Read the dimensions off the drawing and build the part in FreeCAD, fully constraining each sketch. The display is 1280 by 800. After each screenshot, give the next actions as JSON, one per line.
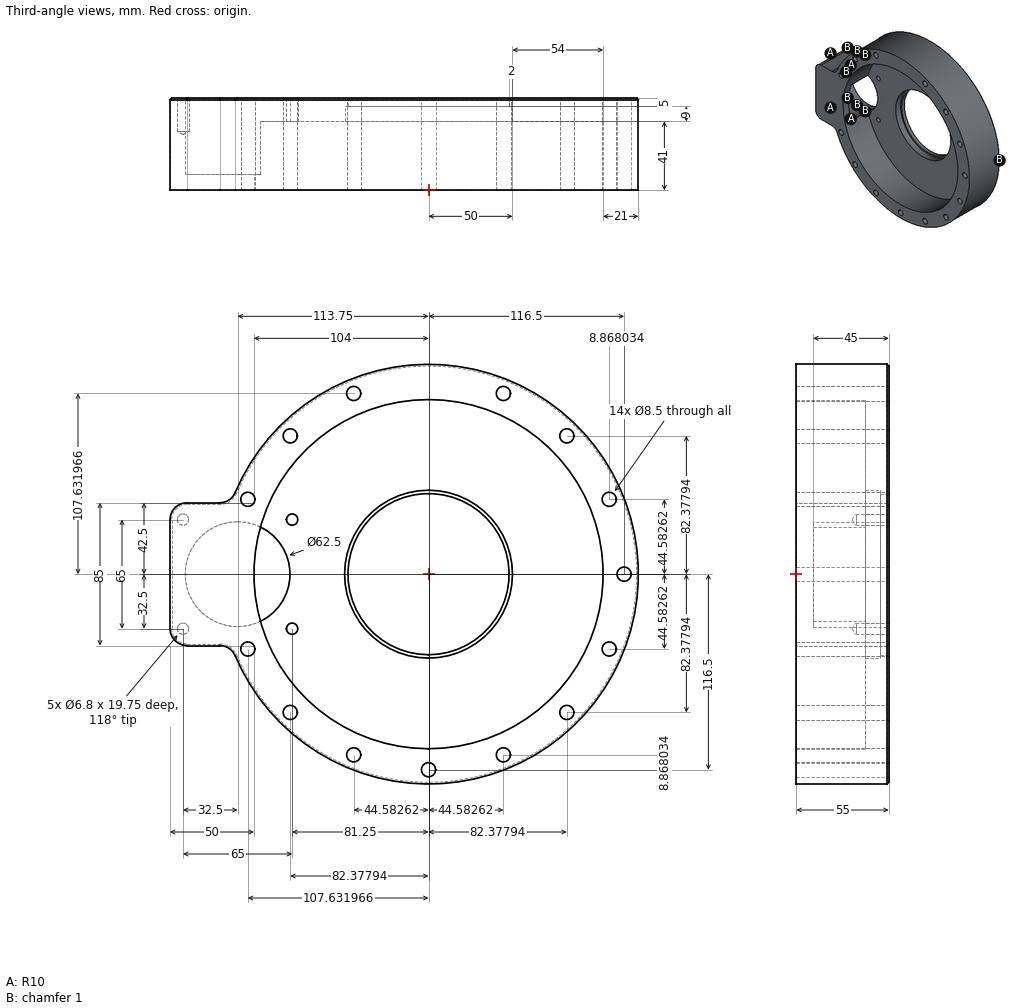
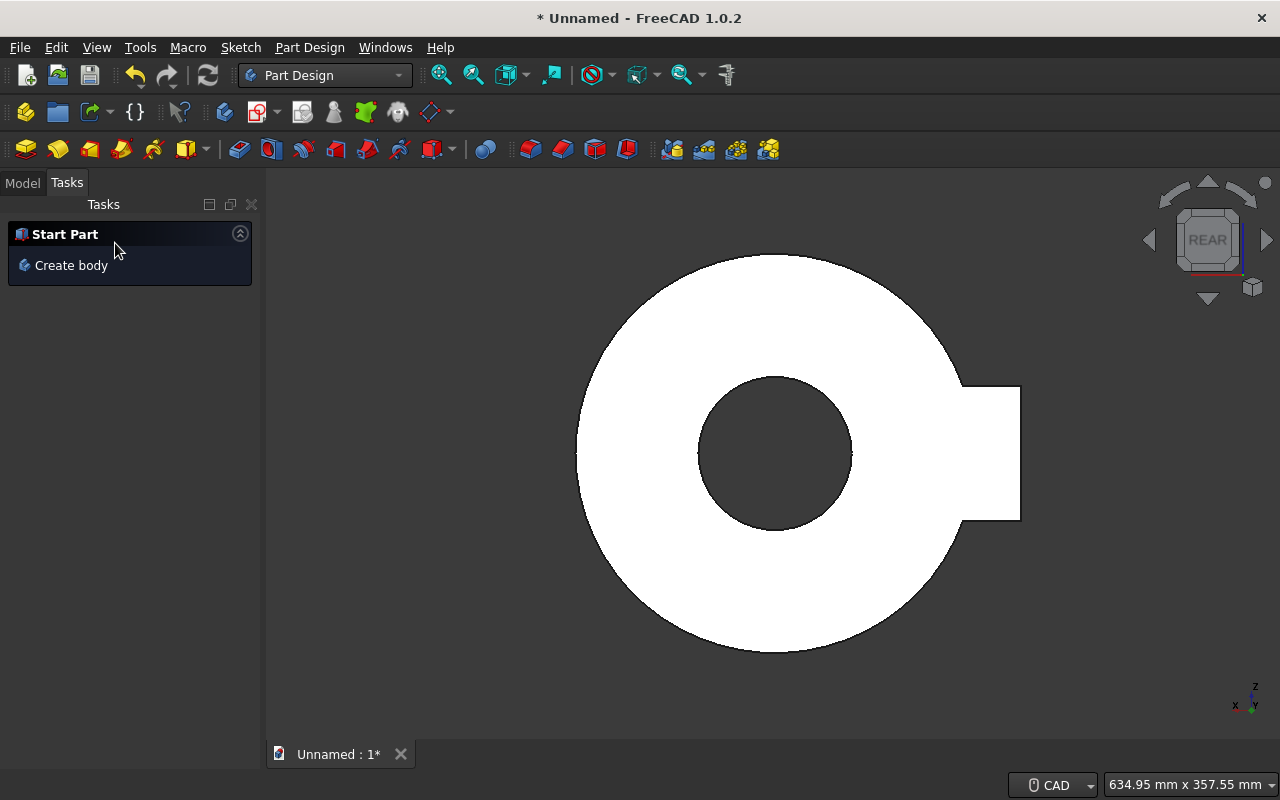
{"action": "left_click", "coordinate": [926, 453]}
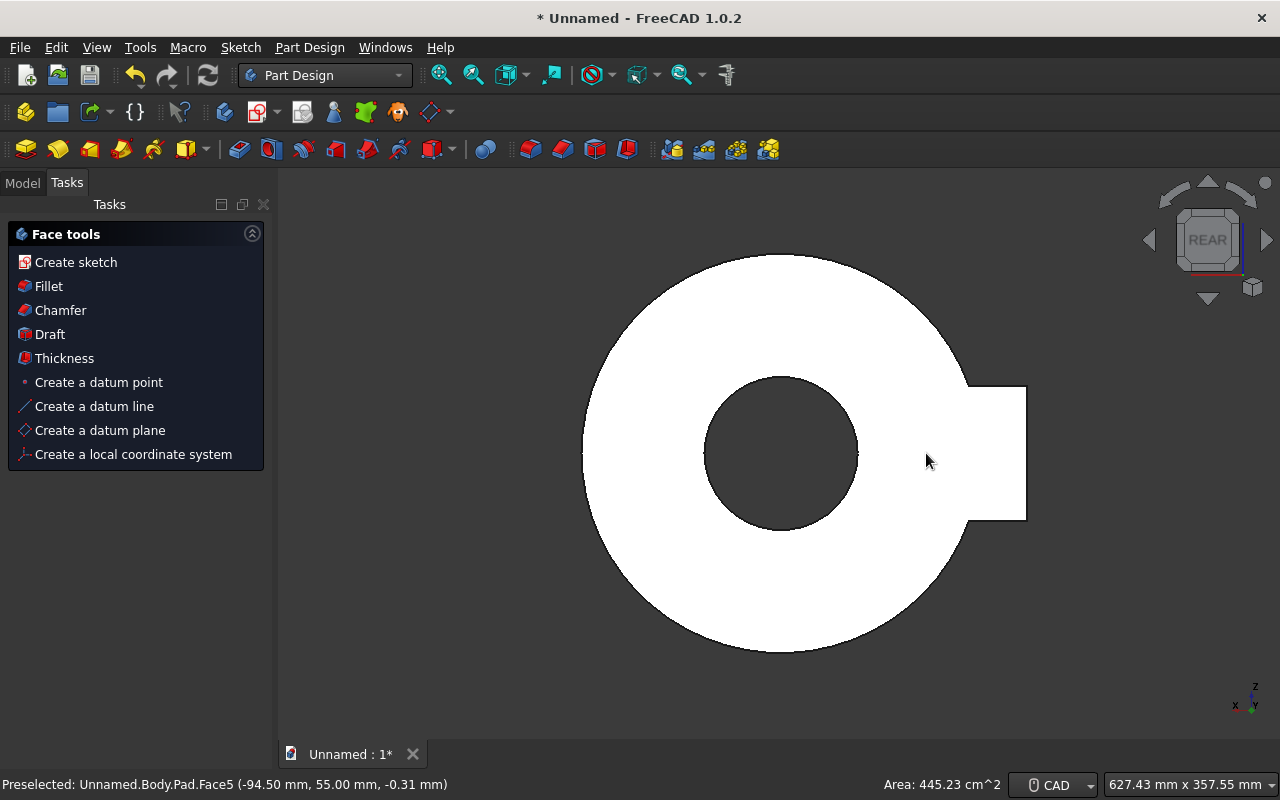
{"action": "left_click", "coordinate": [258, 112]}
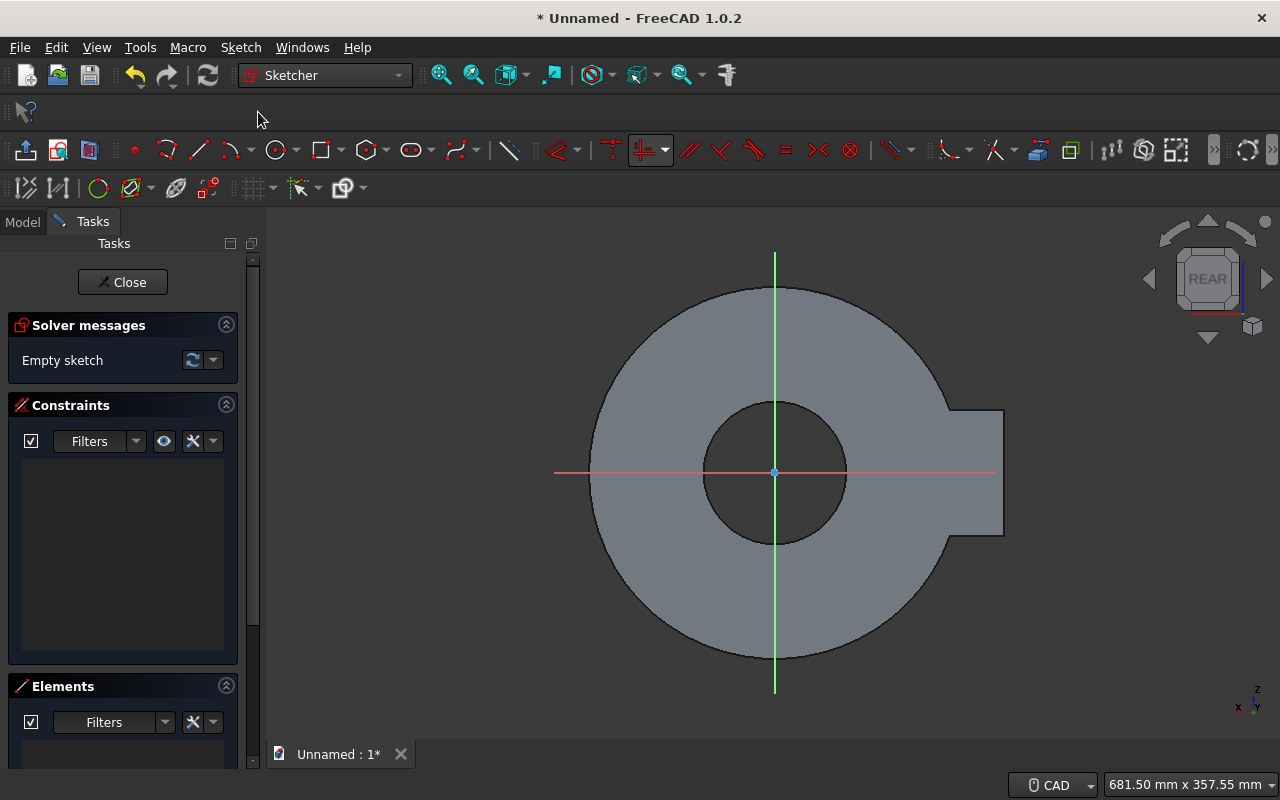
{"action": "scroll", "coordinate": [987, 473], "scroll_direction": "up", "scroll_amount": 5}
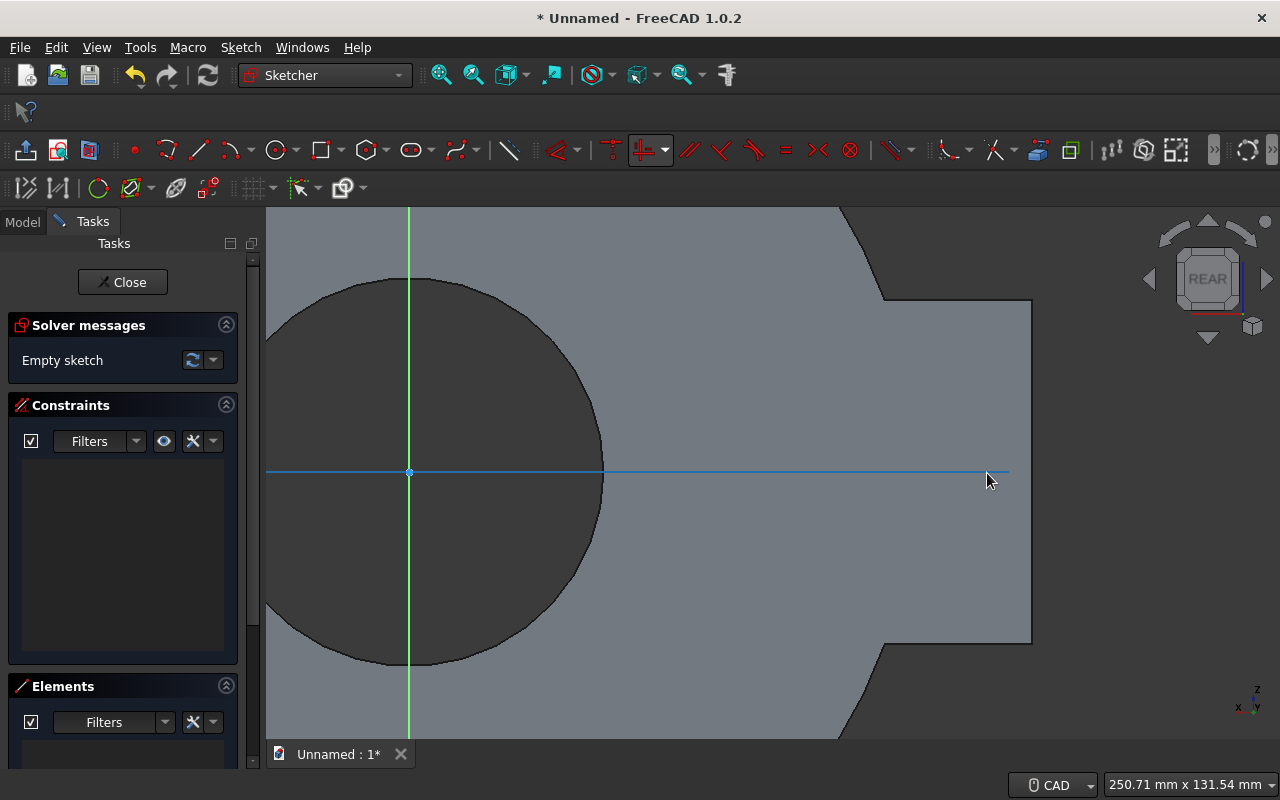
{"action": "left_click", "coordinate": [276, 150]}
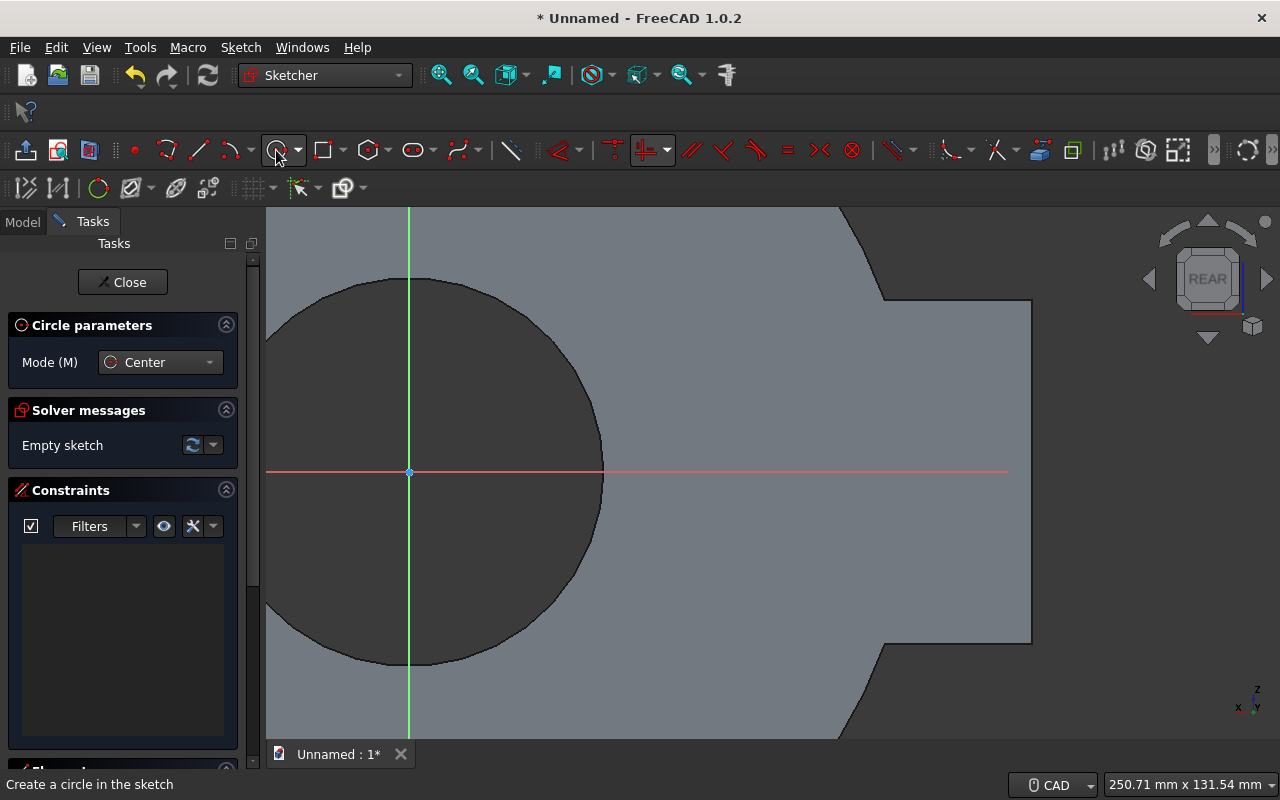
{"action": "left_click", "coordinate": [869, 472]}
{"action": "left_click", "coordinate": [959, 383]}
{"action": "key", "text": "Escape"}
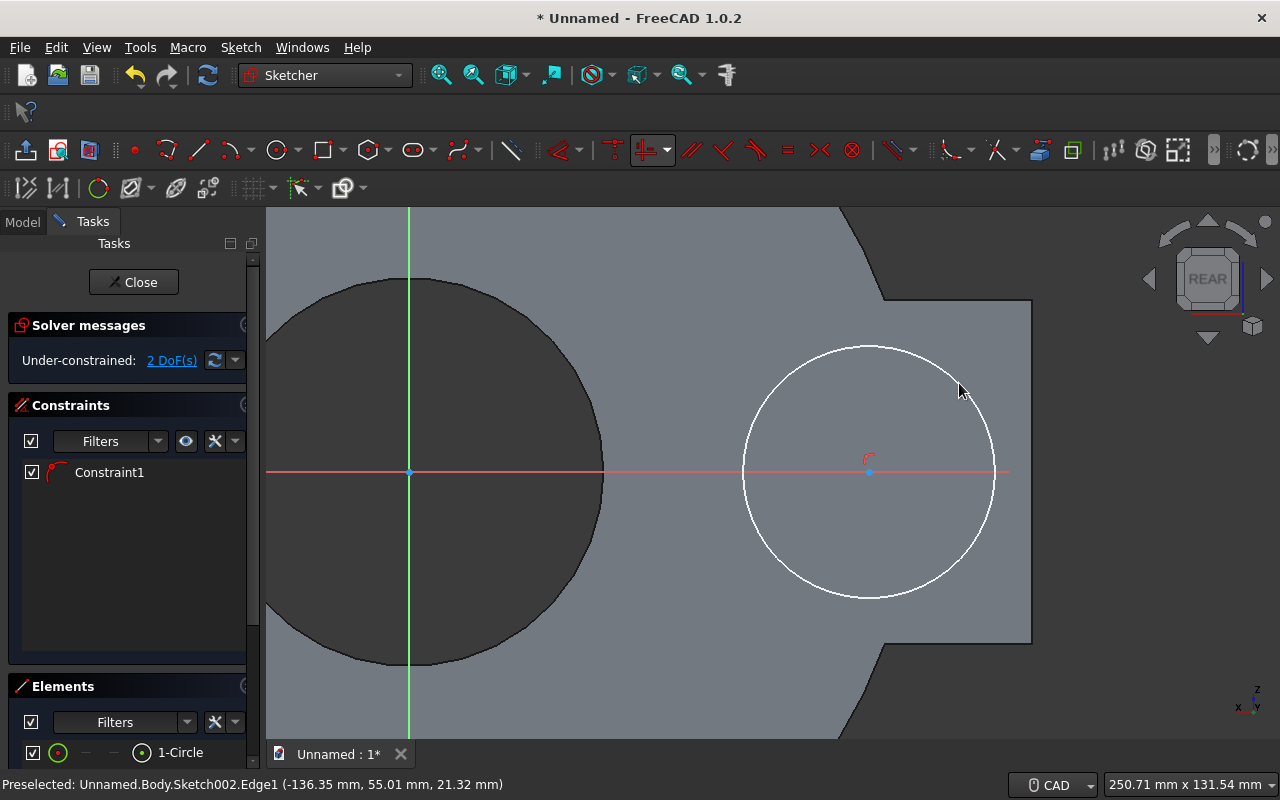
{"action": "left_click", "coordinate": [558, 150]}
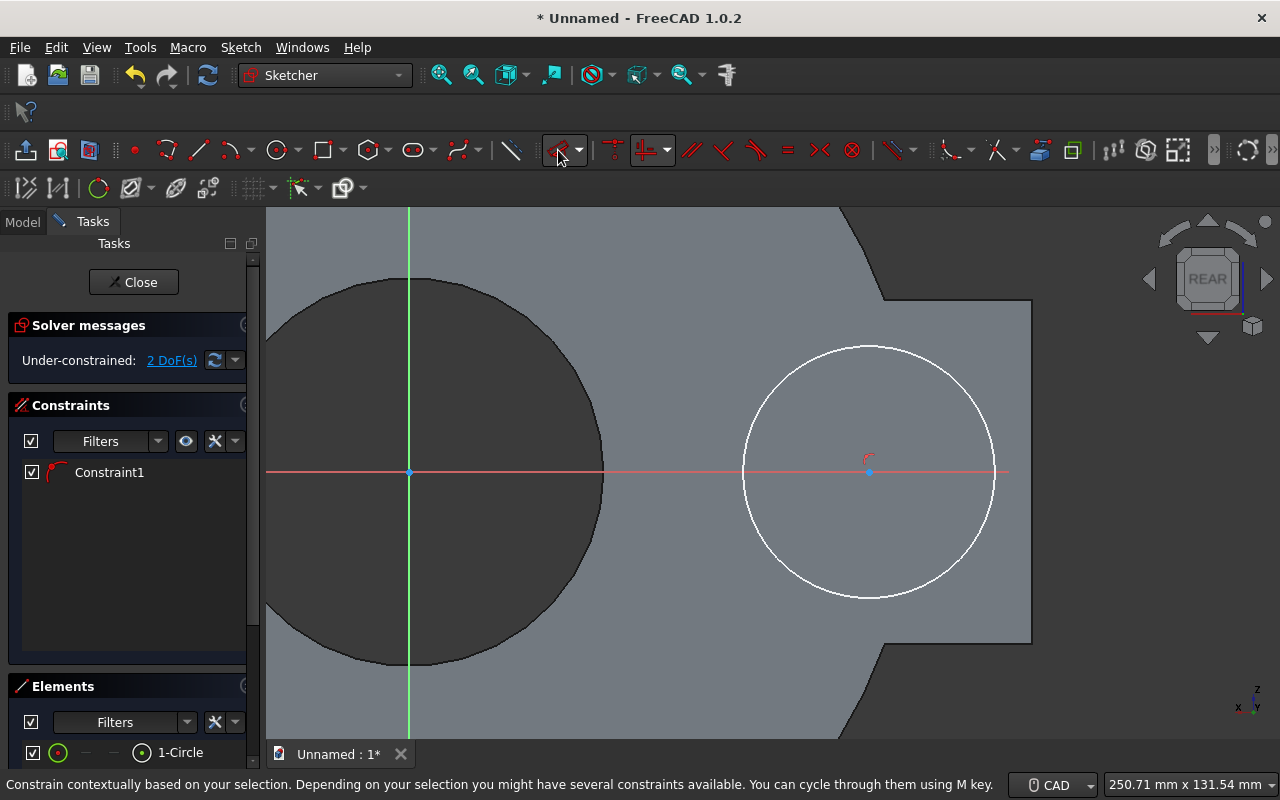
{"action": "left_click", "coordinate": [958, 383]}
{"action": "left_click", "coordinate": [981, 360]}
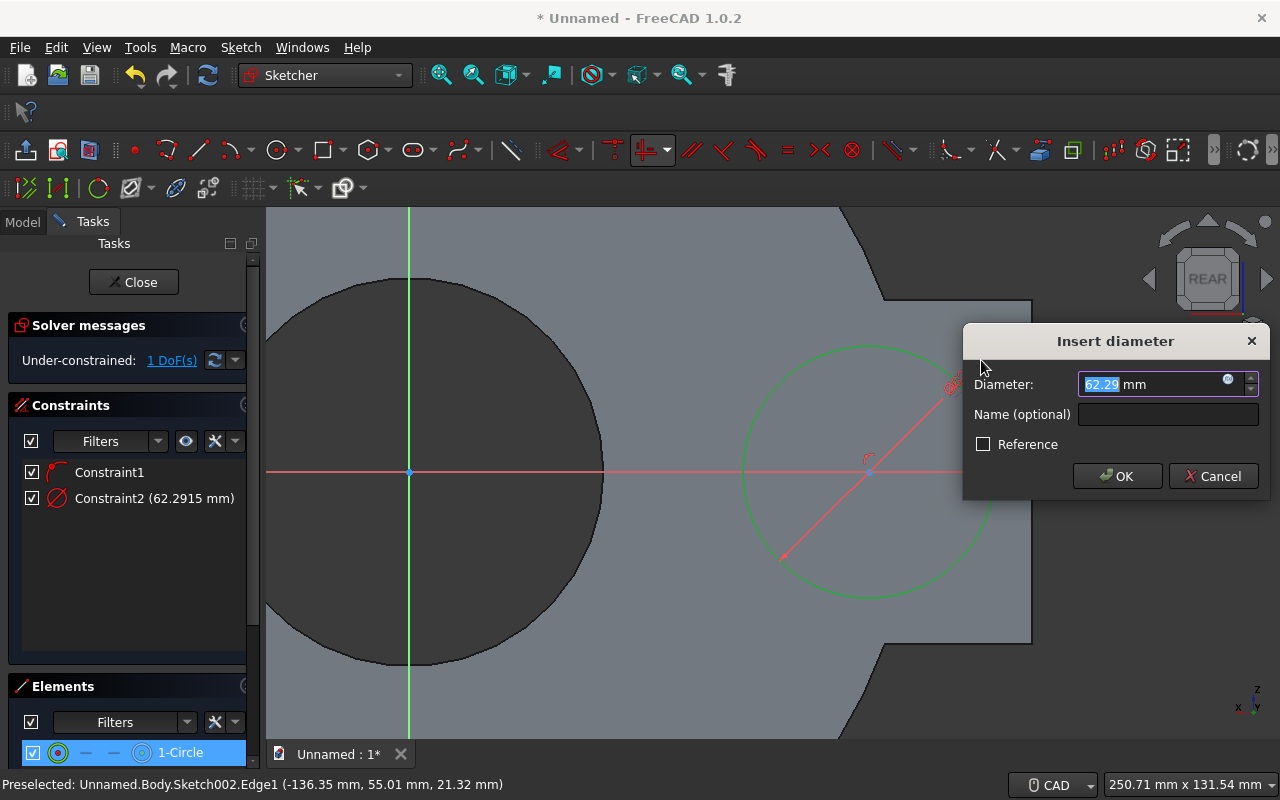
{"action": "type", "text": "62.5"}
{"action": "key", "text": "Return"}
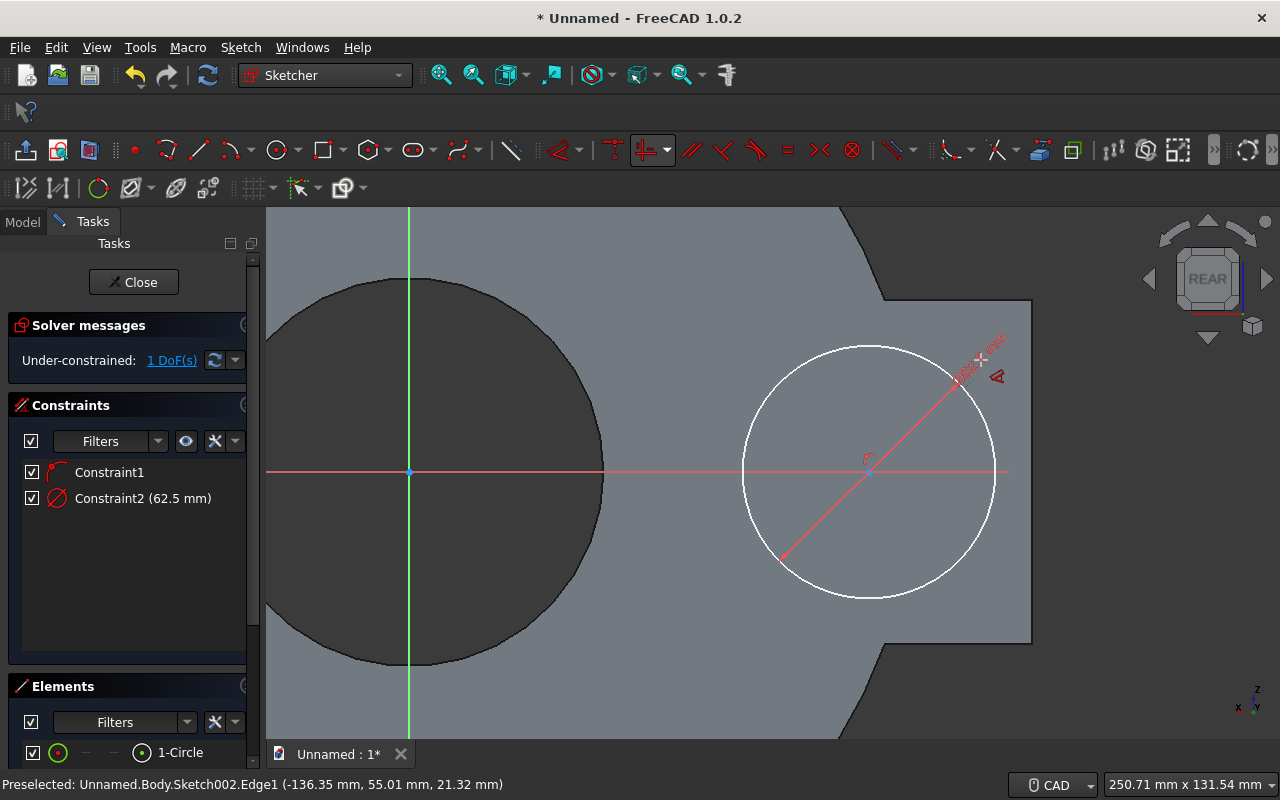
{"action": "left_click", "coordinate": [869, 472]}
{"action": "left_click", "coordinate": [639, 506]}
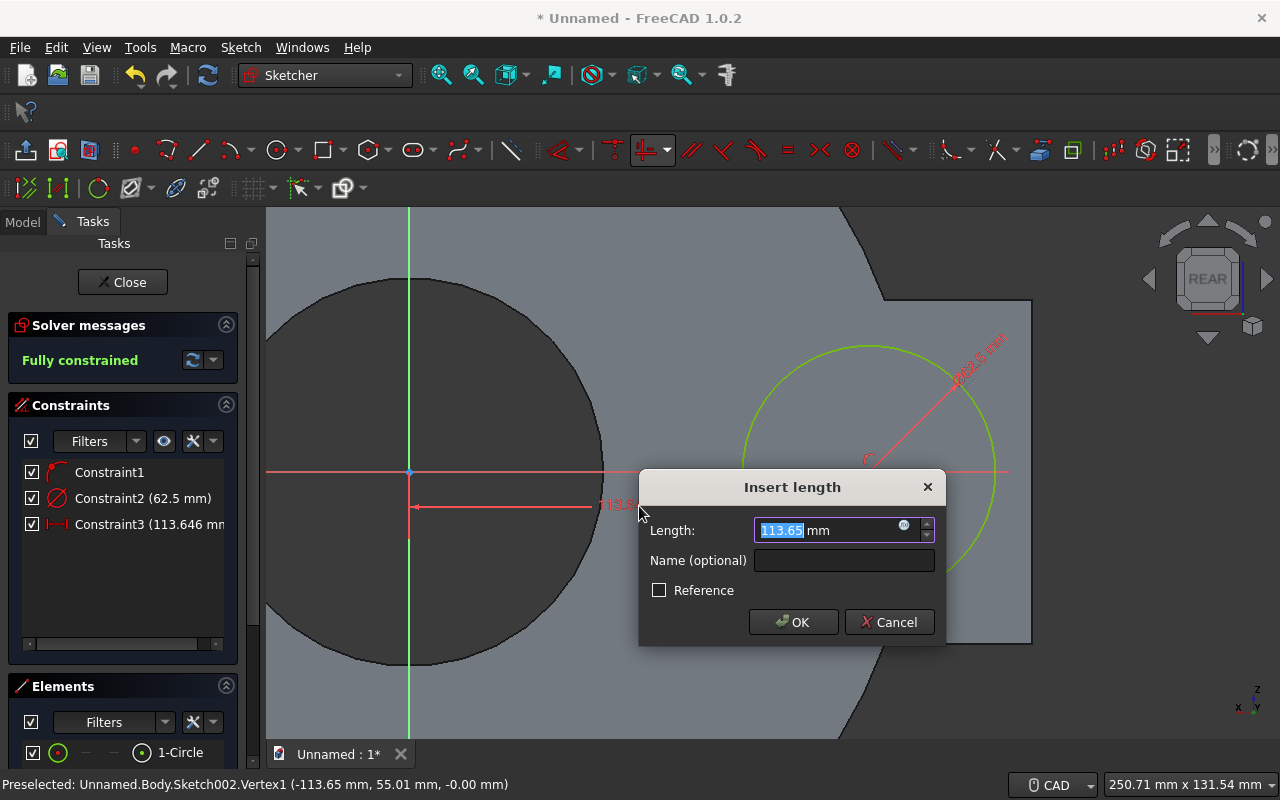
{"action": "type", "text": "113.75"}
{"action": "key", "text": "Return"}
{"action": "key", "text": "Escape"}